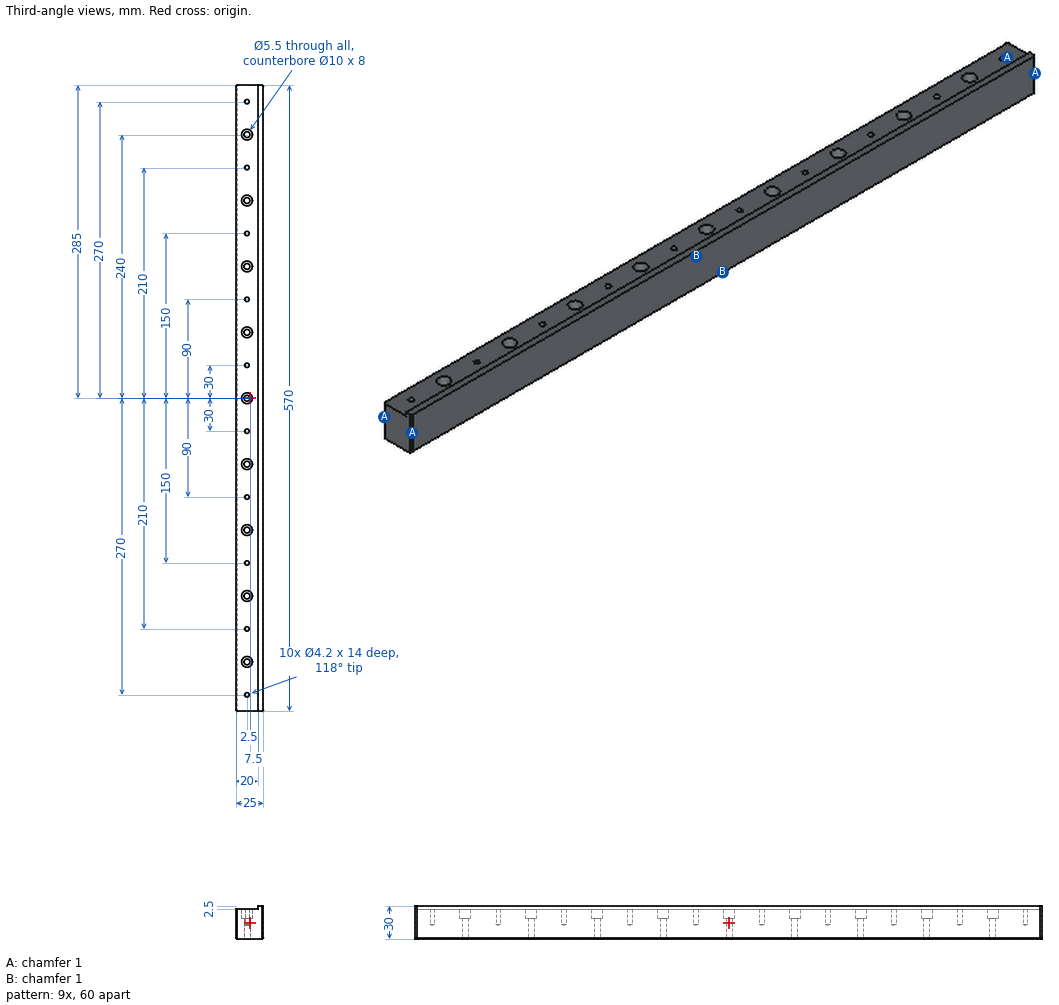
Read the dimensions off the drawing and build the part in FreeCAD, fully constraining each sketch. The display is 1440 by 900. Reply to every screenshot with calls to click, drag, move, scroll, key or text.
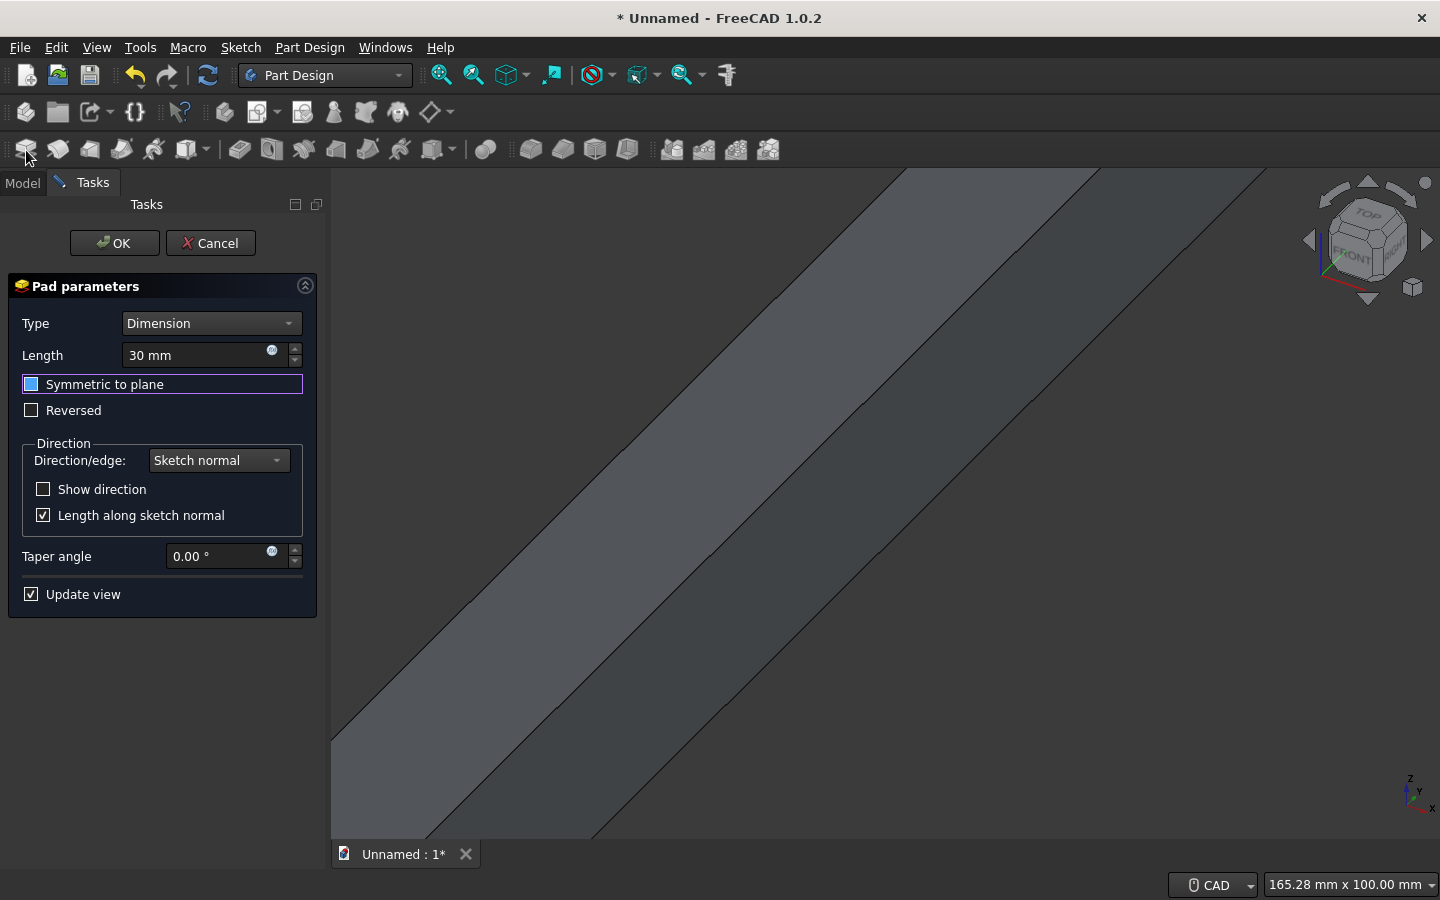
click(30, 384)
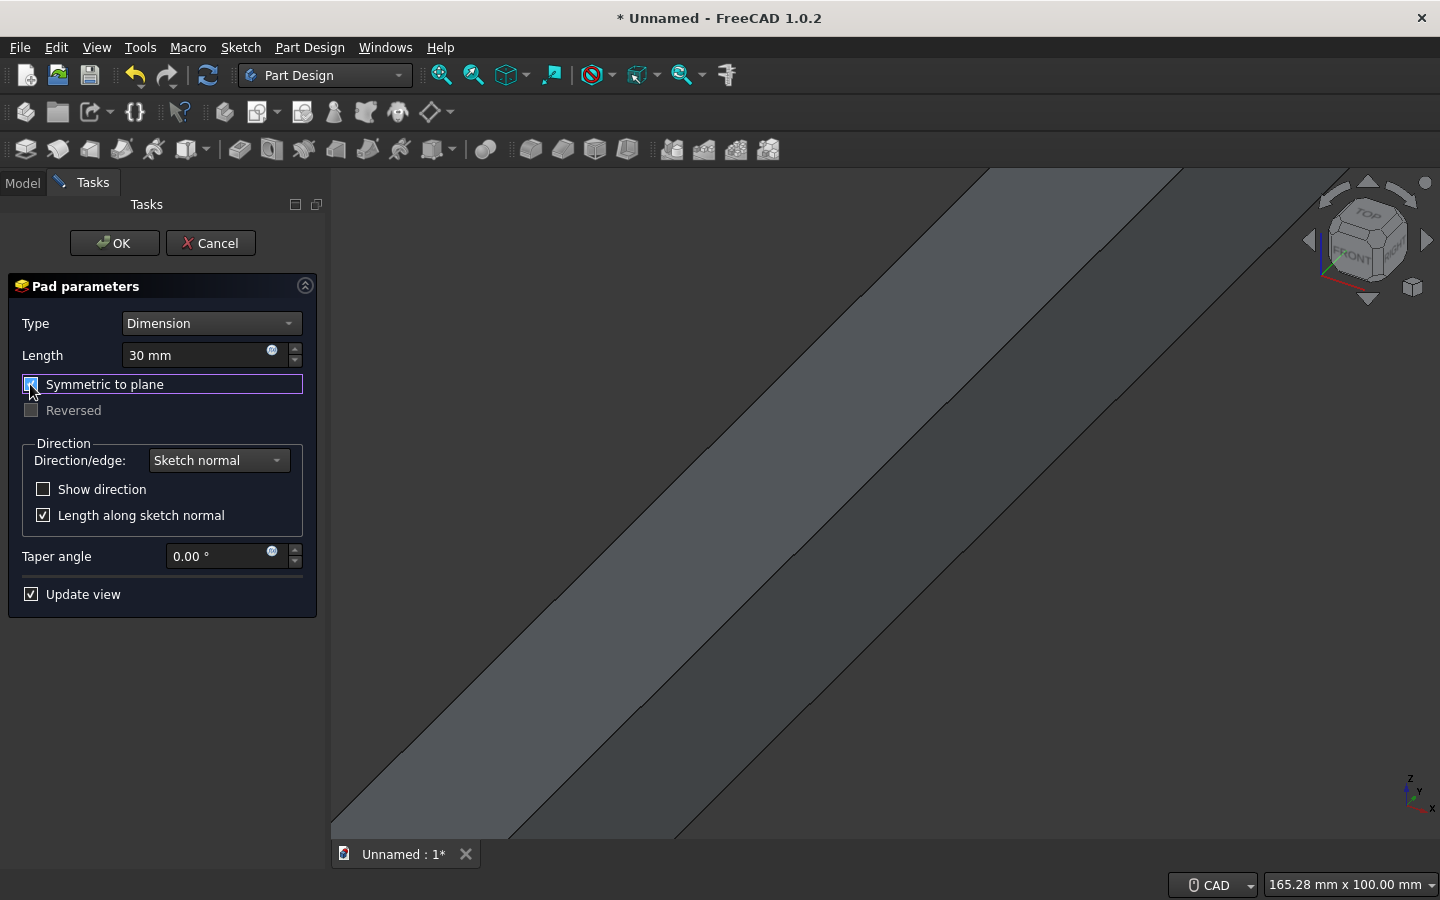
click(115, 243)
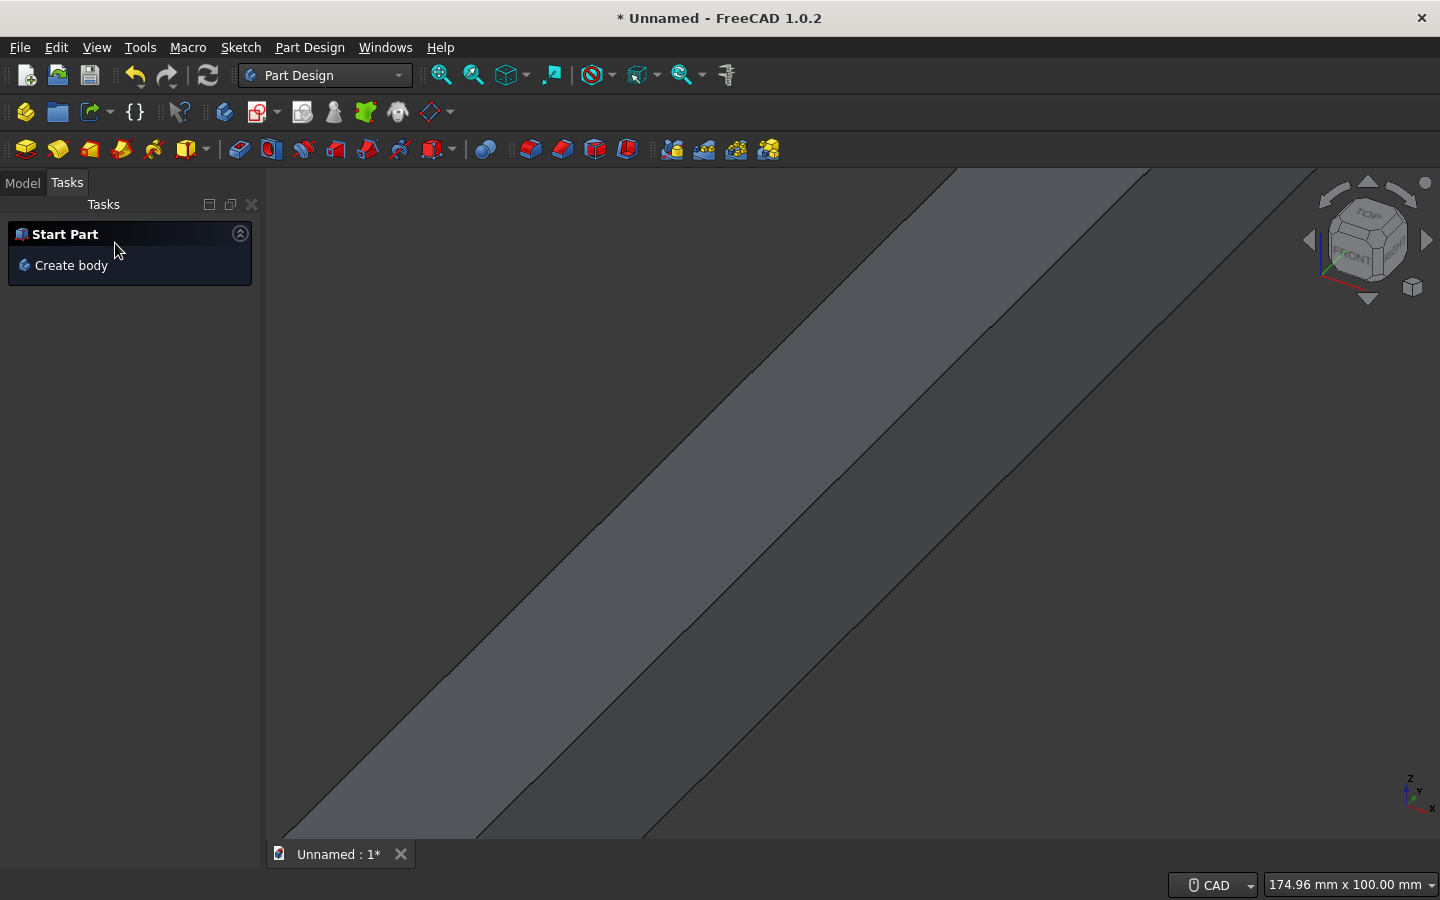
click(442, 76)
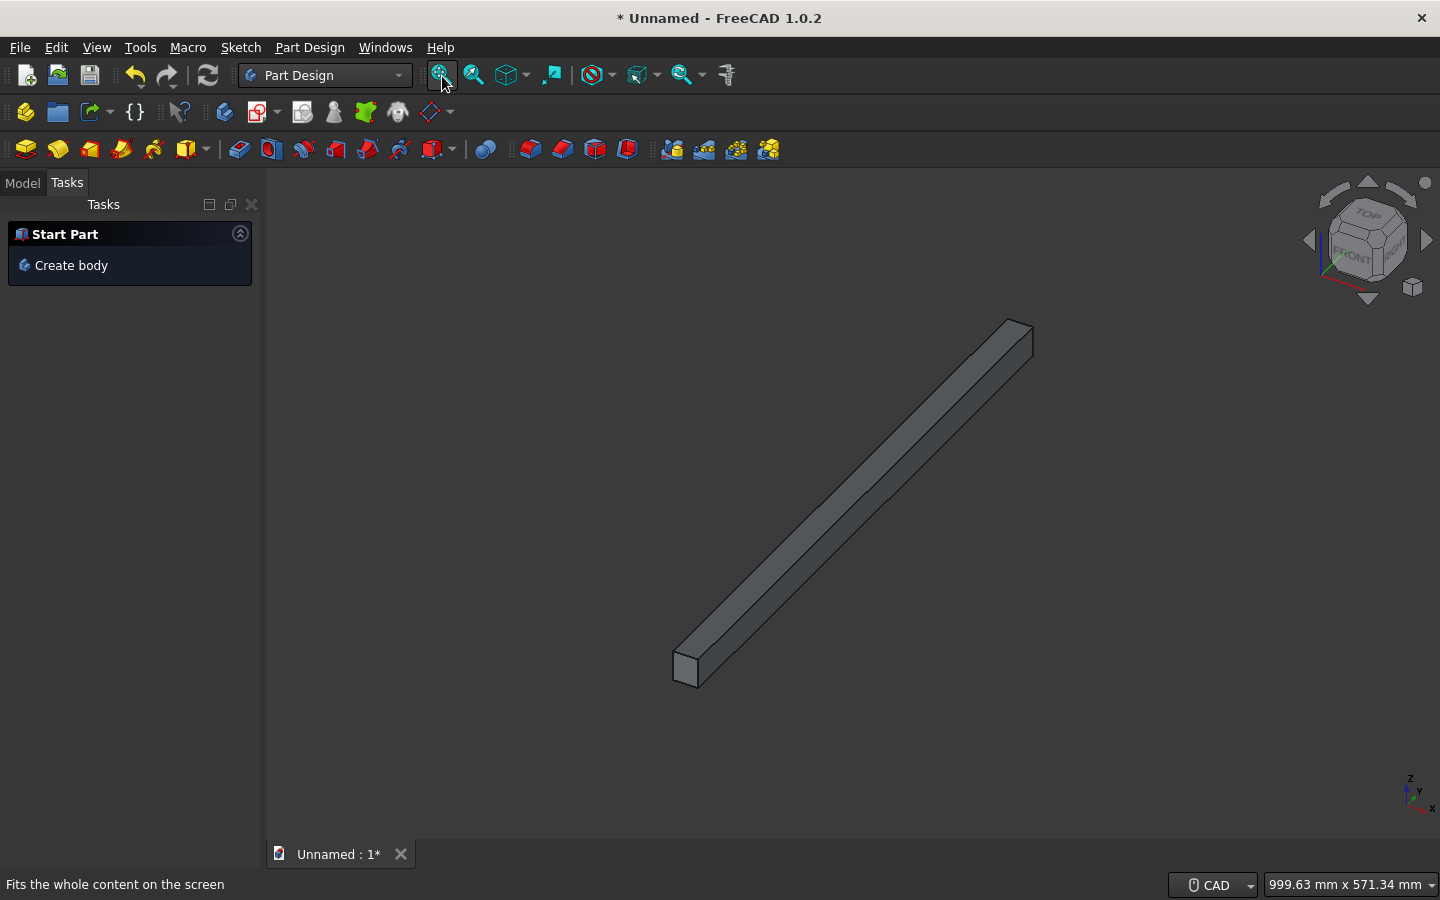
click(698, 673)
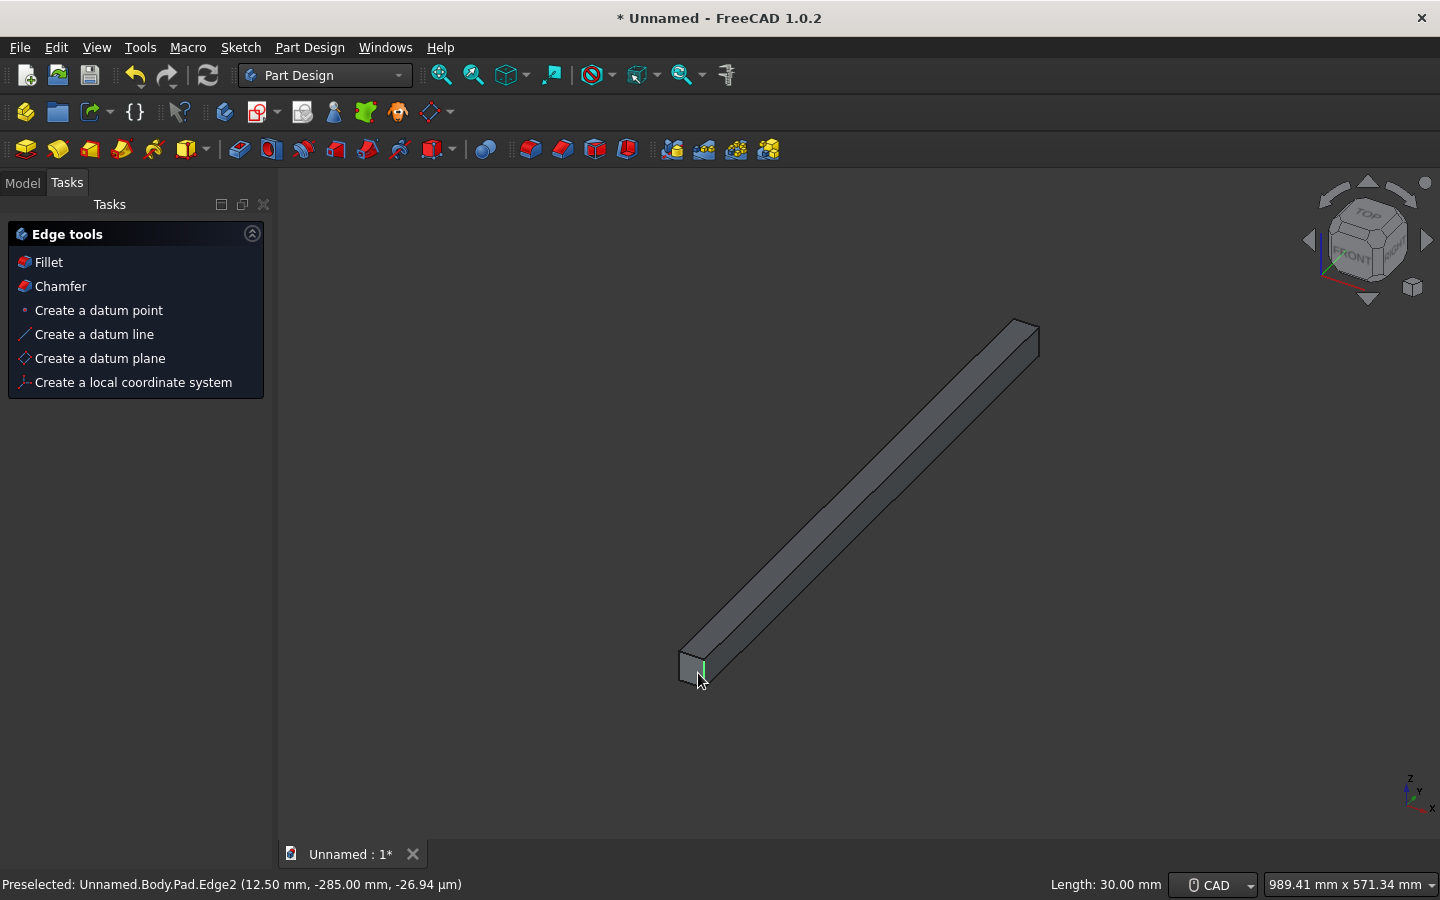
key(0)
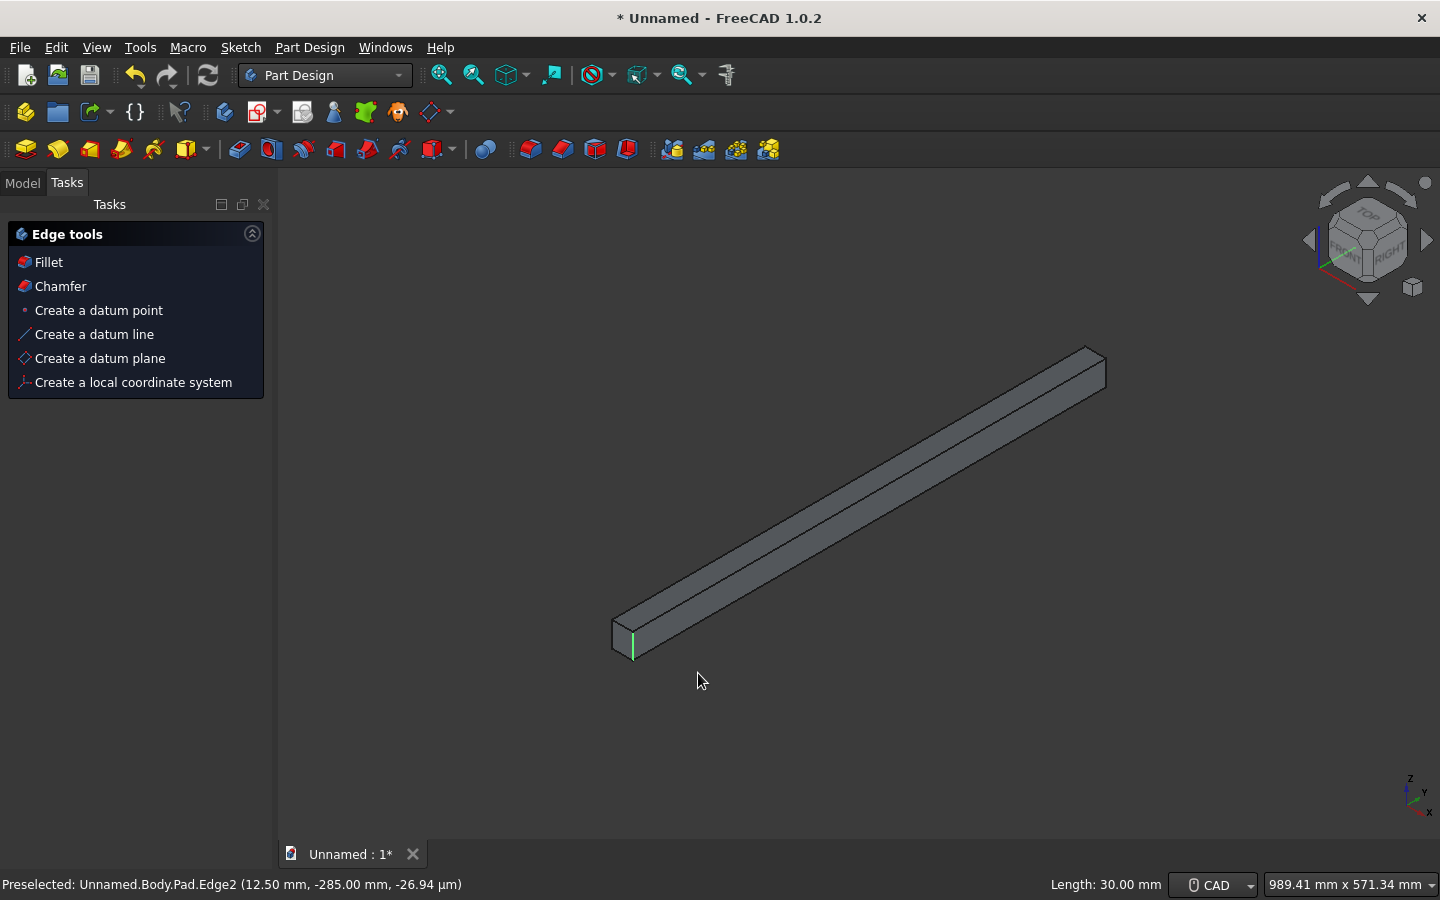
key(2)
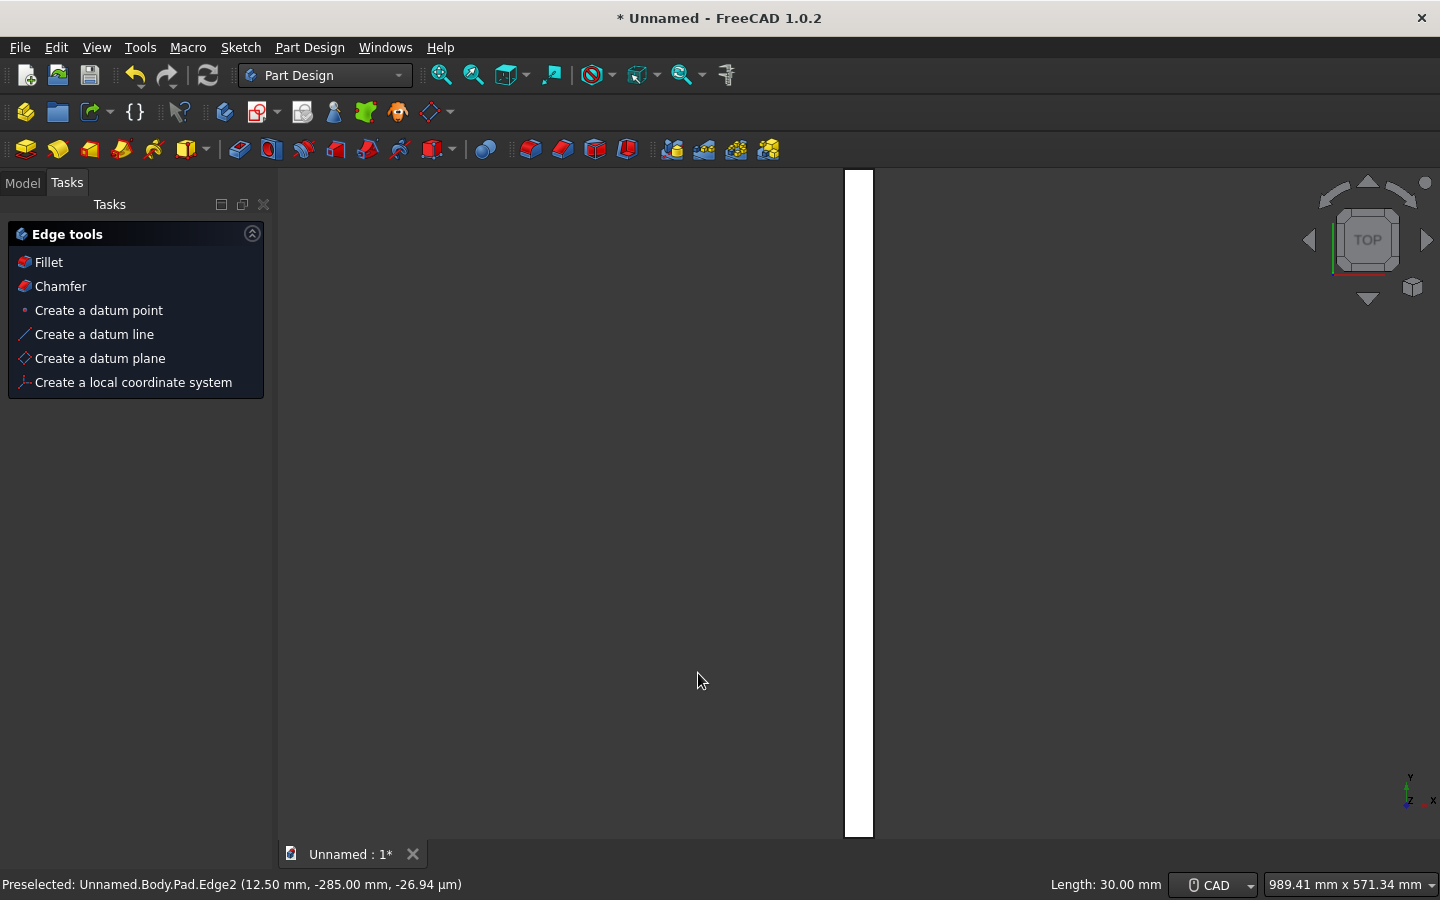
key(1)